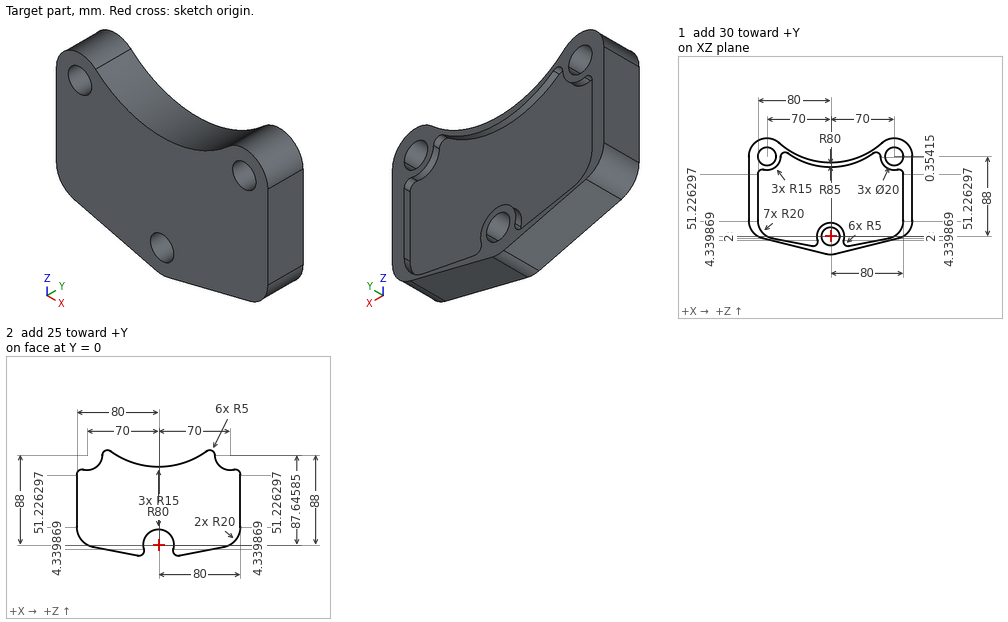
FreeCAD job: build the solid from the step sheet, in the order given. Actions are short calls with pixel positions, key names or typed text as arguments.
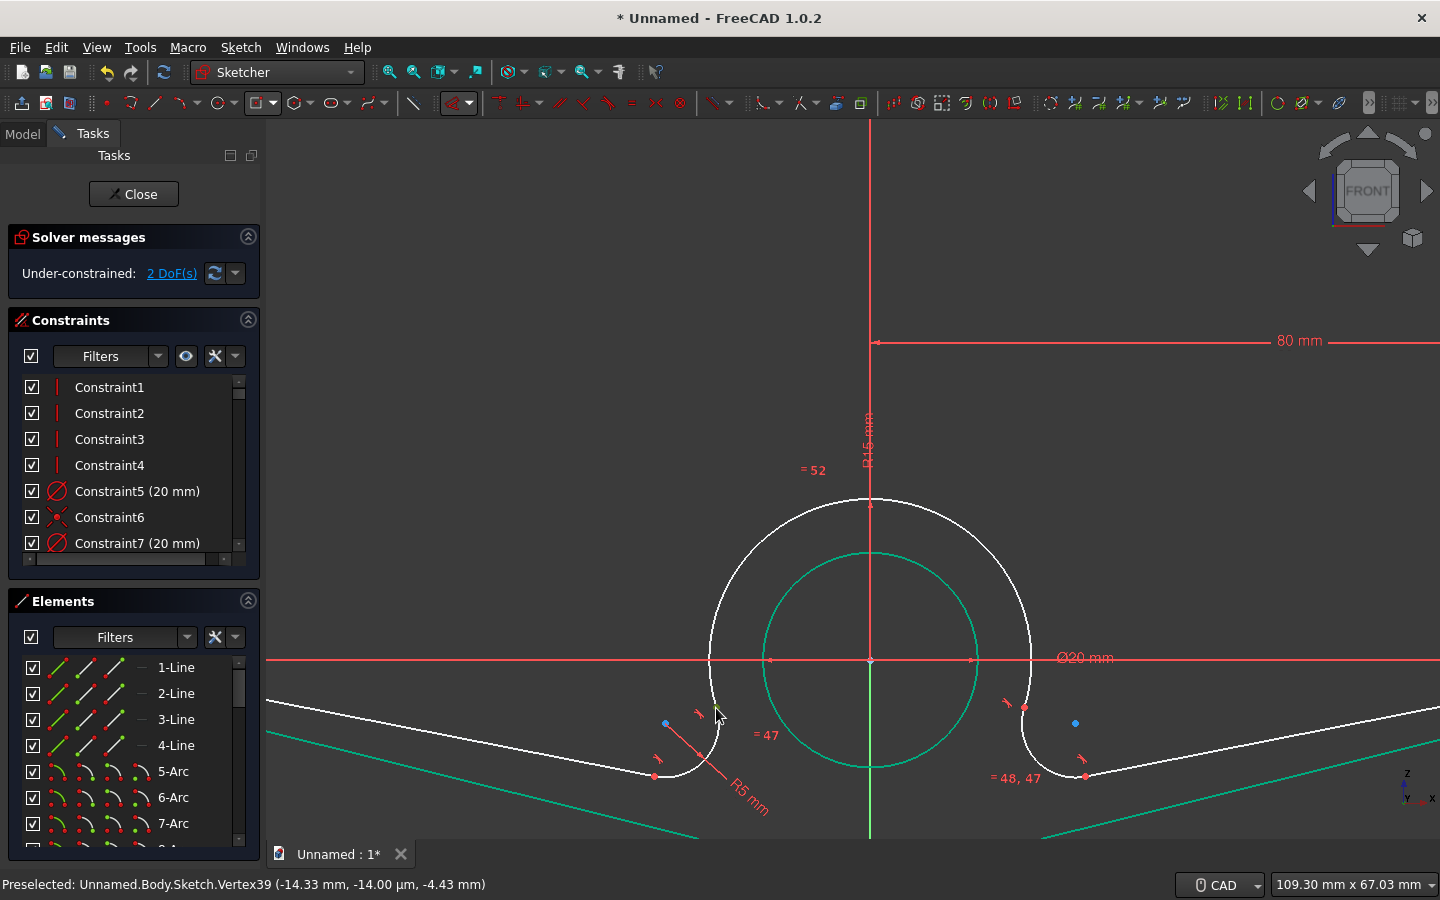
key(i)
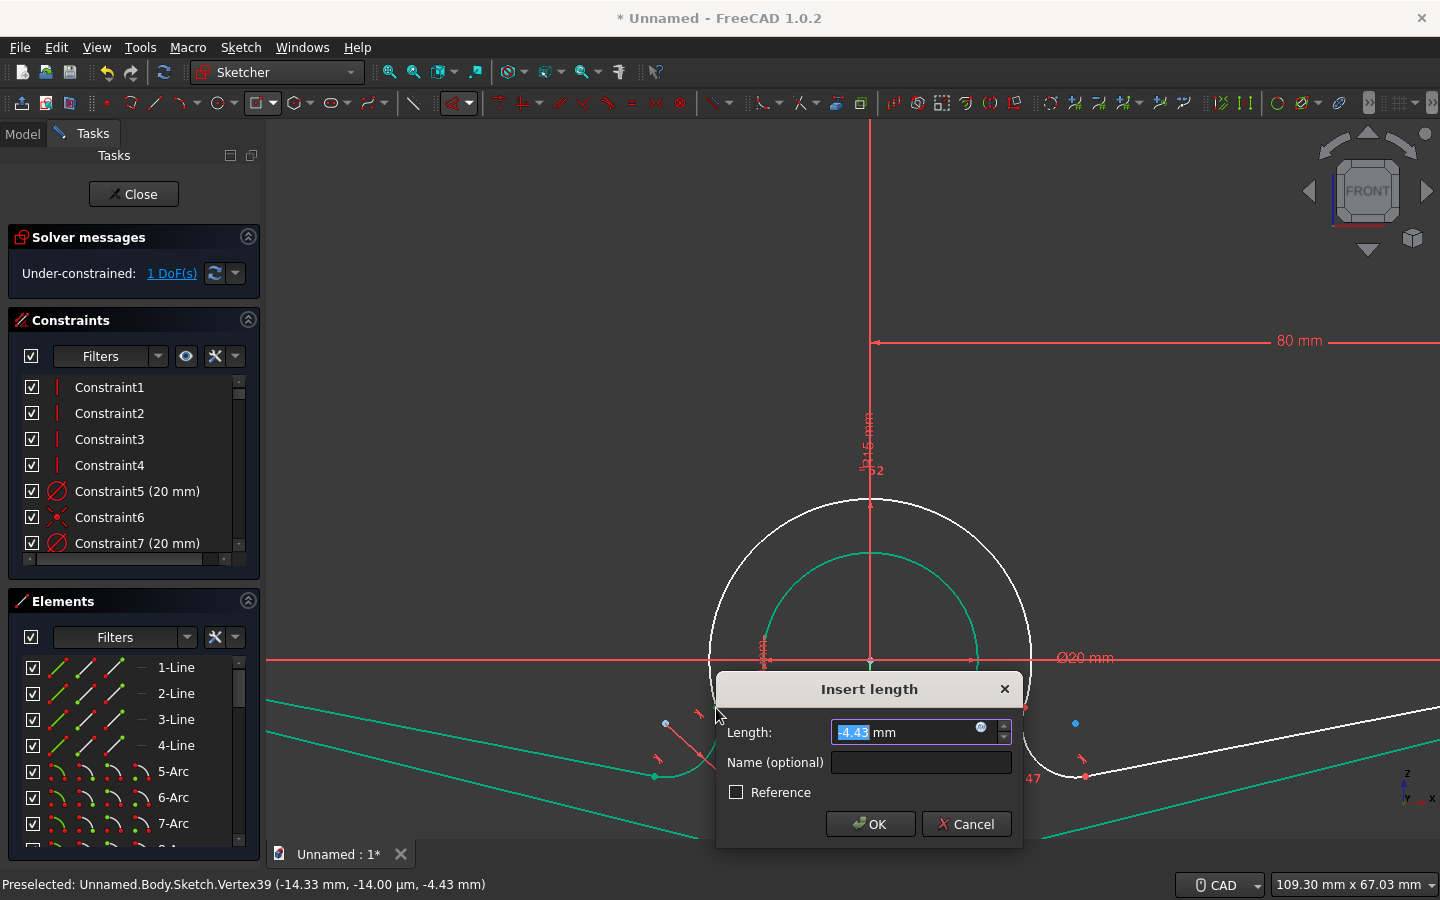
text(-4.339869)
key(Return)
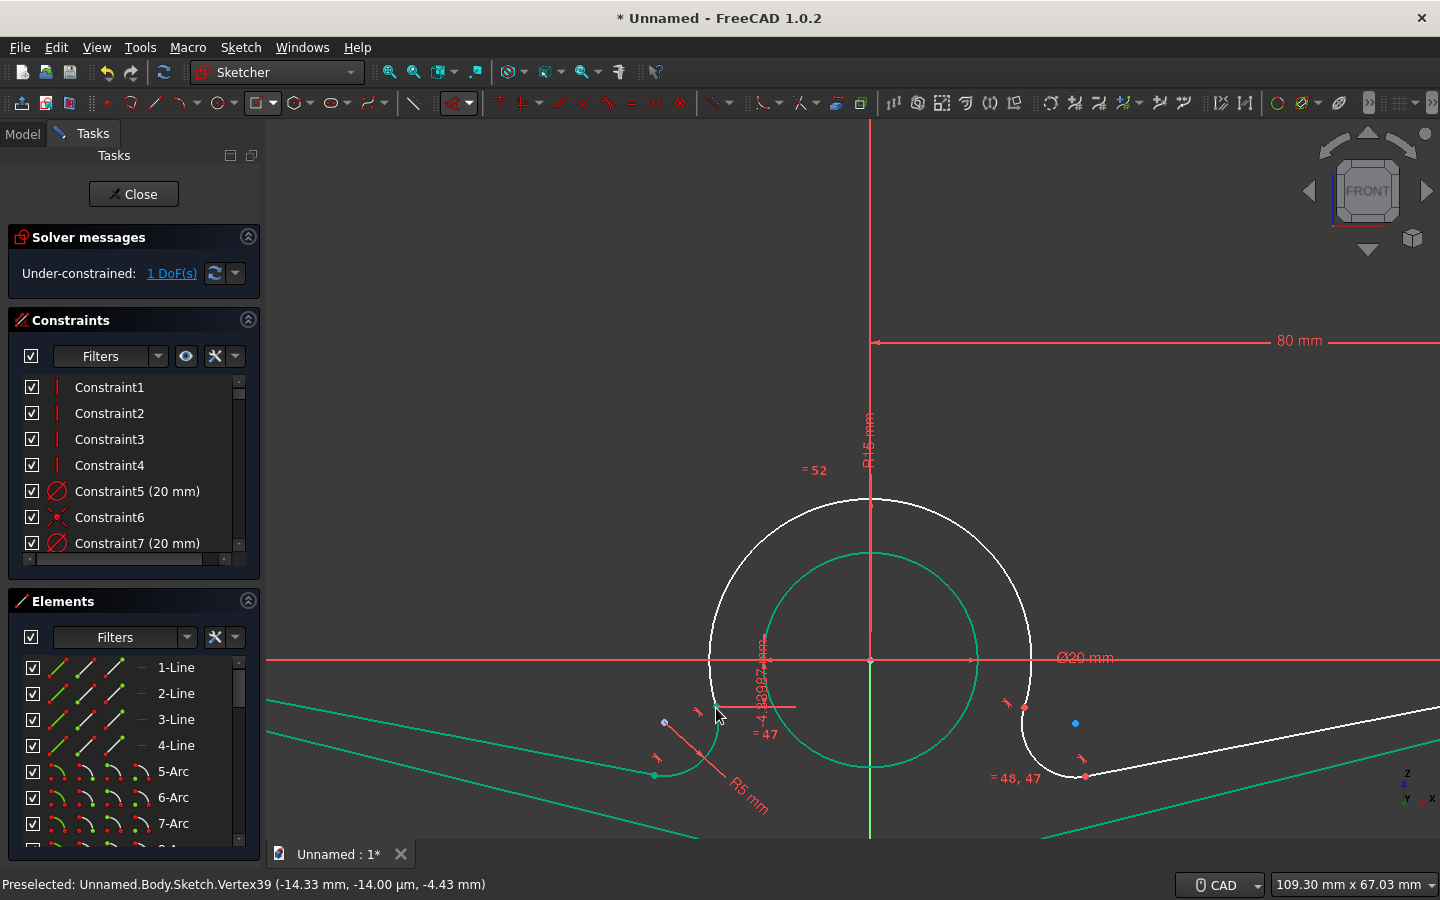
click(1024, 708)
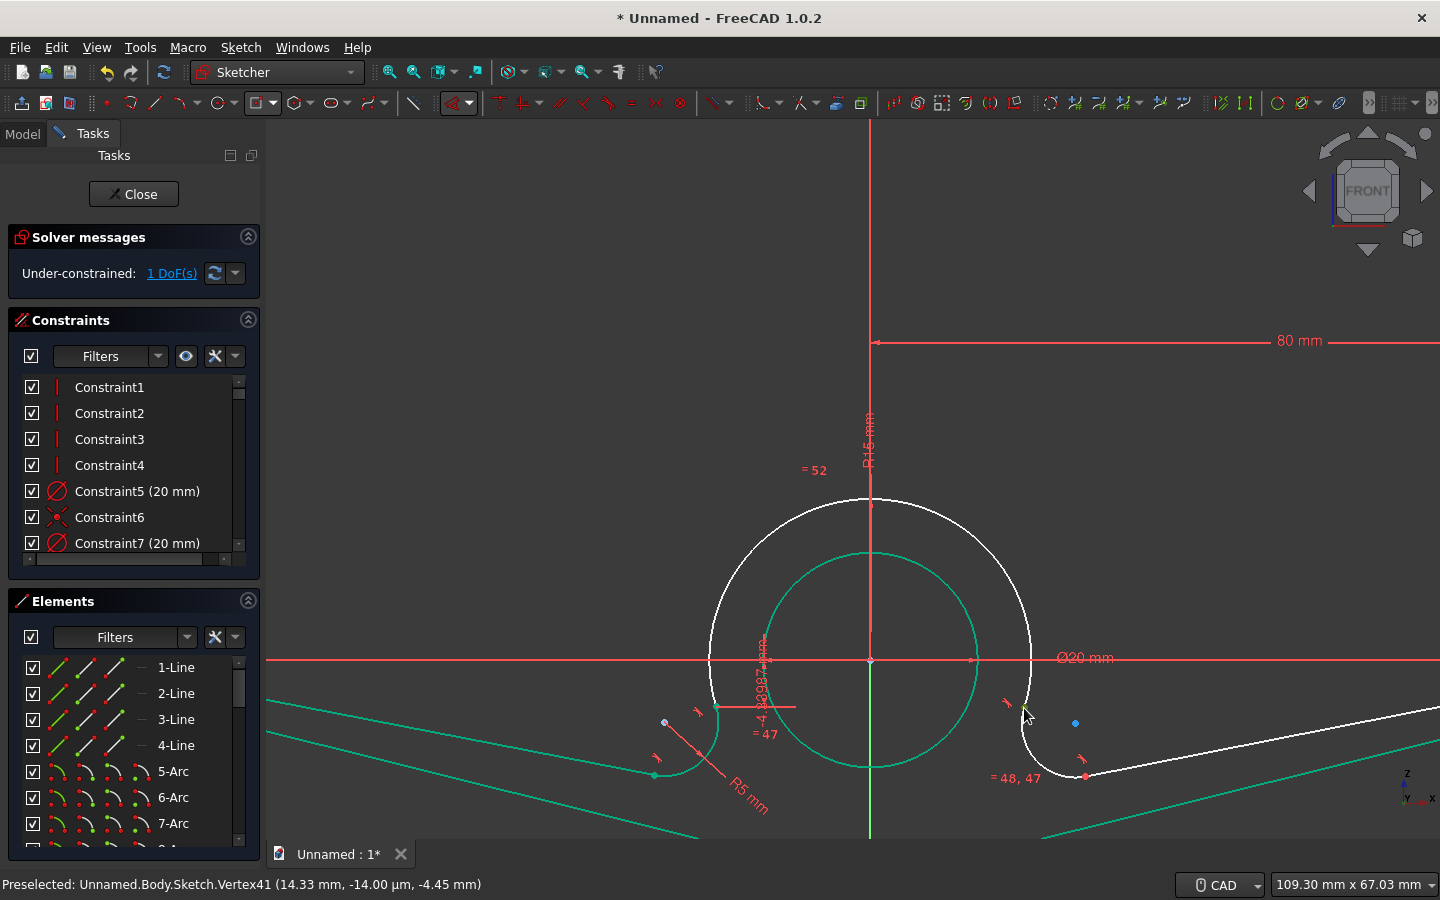
key(i)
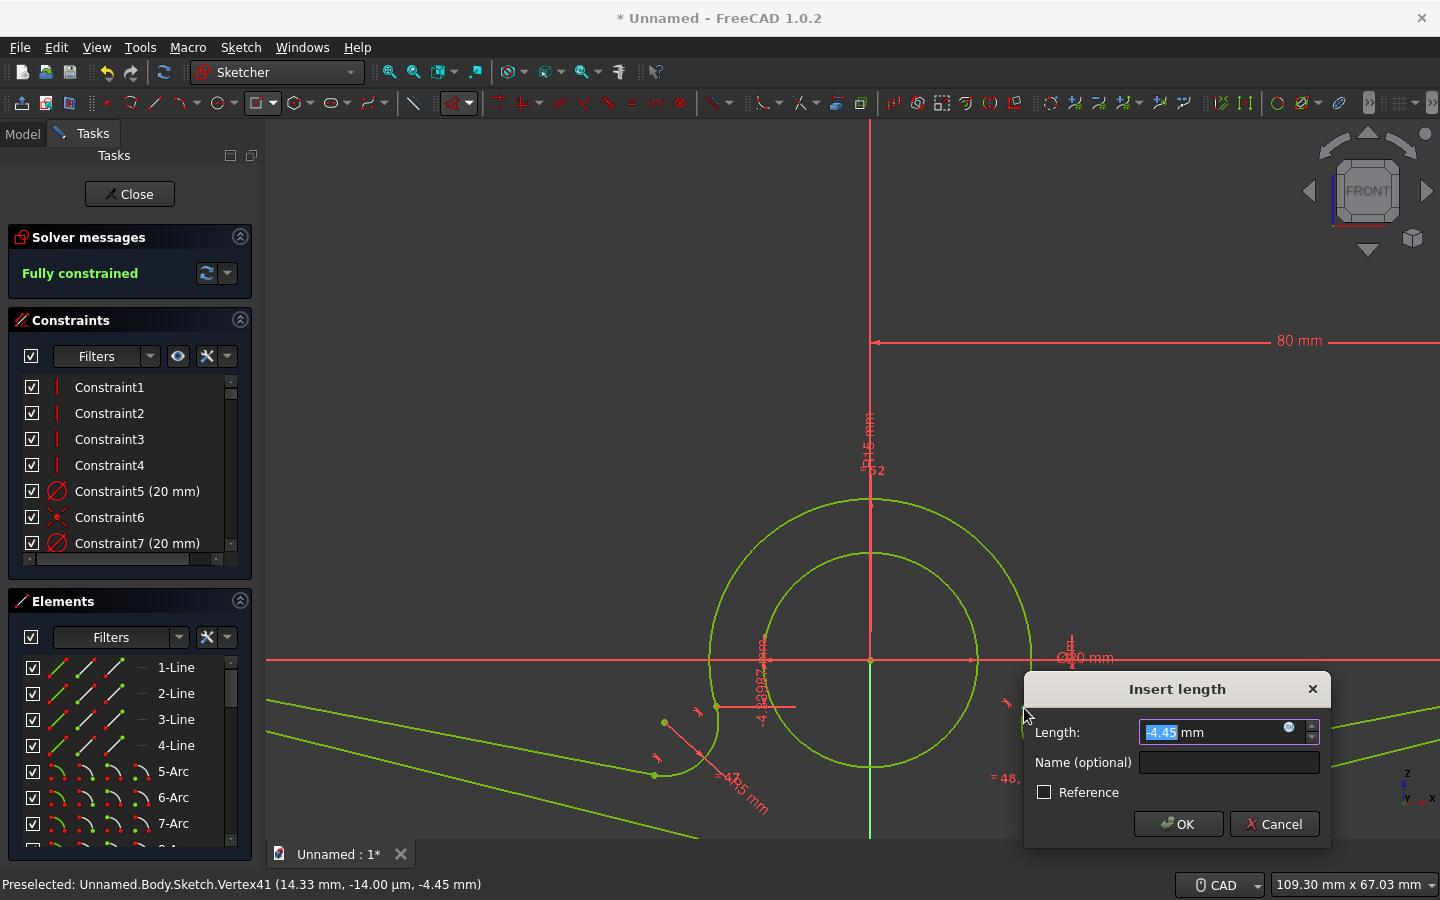
text(-4.339869)
key(Return)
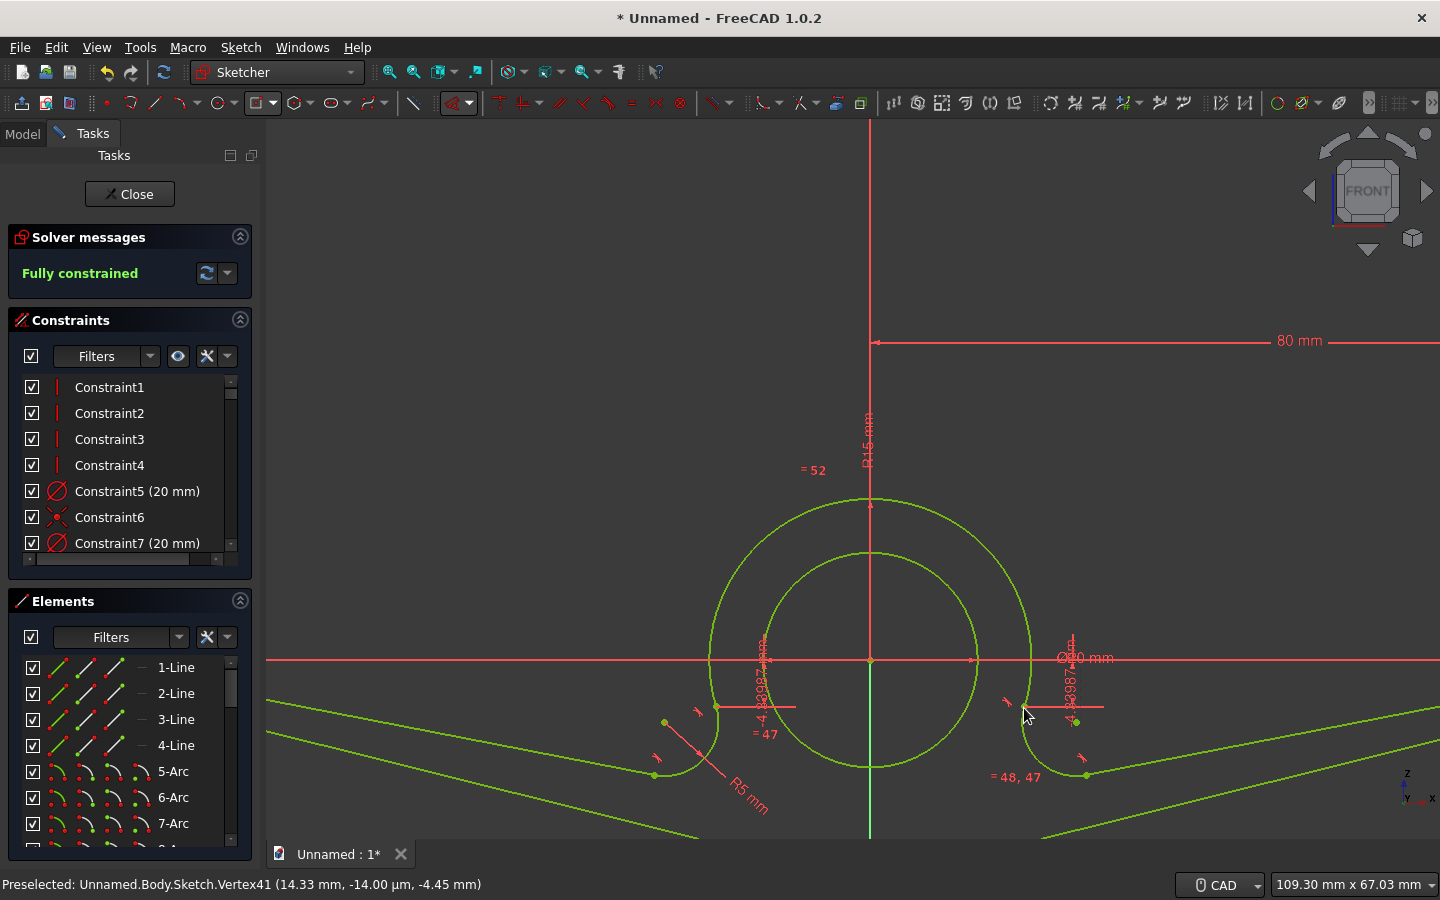
click(130, 194)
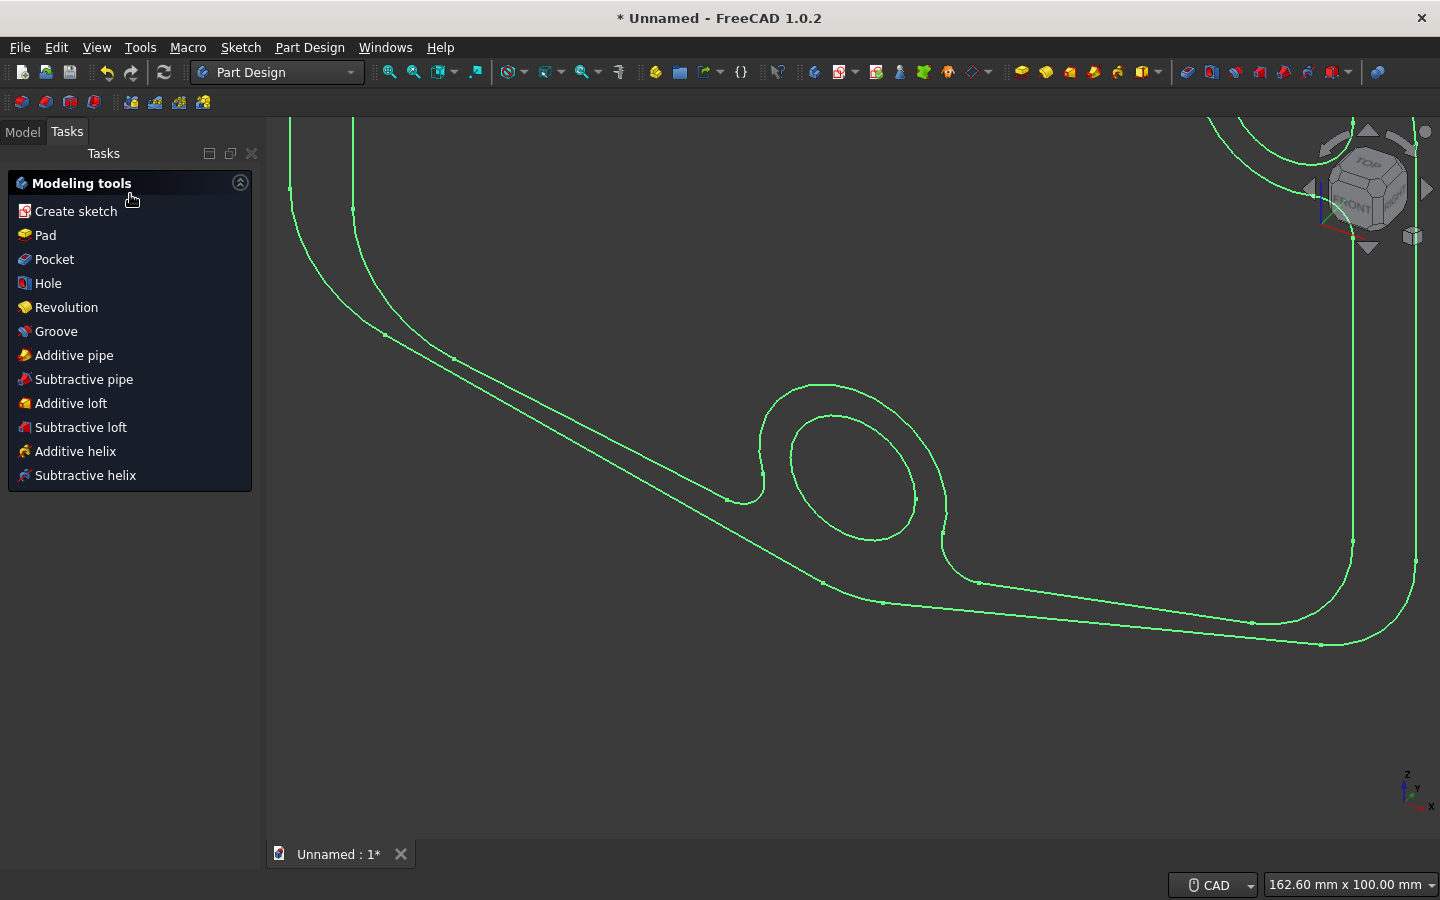
click(1022, 72)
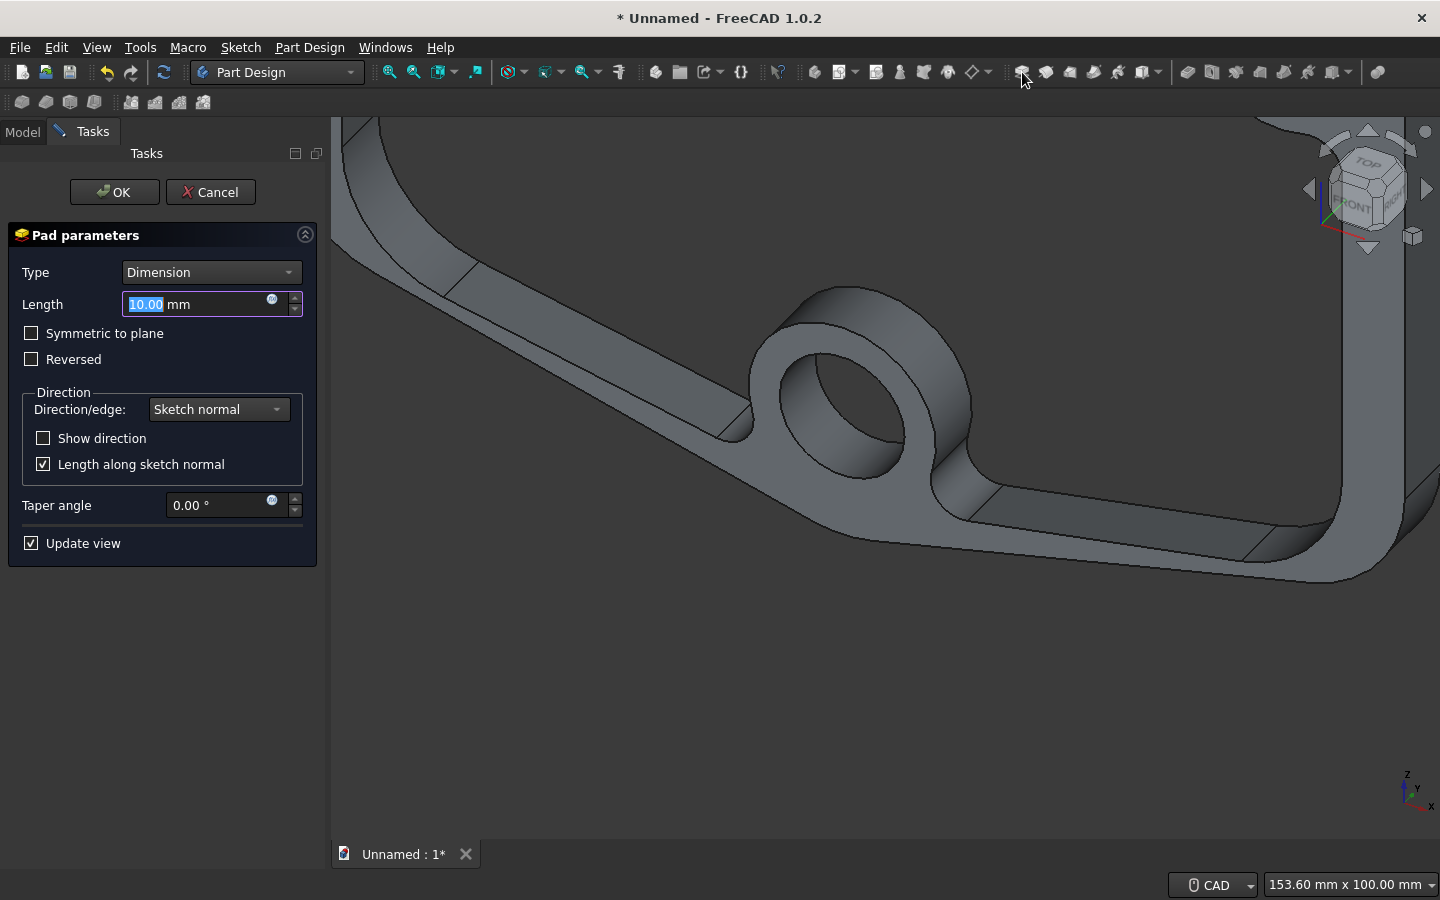
text(30)
key(Tab)